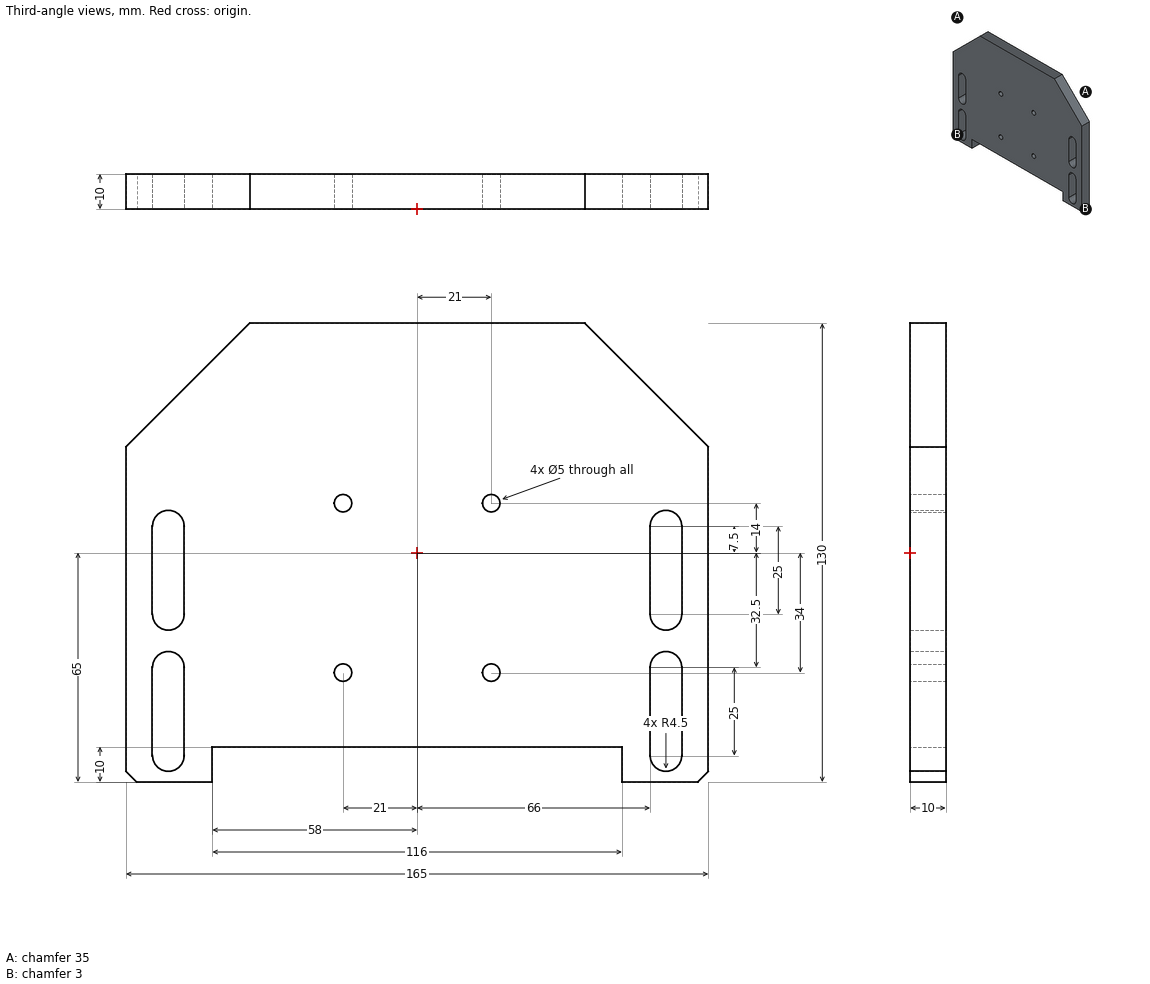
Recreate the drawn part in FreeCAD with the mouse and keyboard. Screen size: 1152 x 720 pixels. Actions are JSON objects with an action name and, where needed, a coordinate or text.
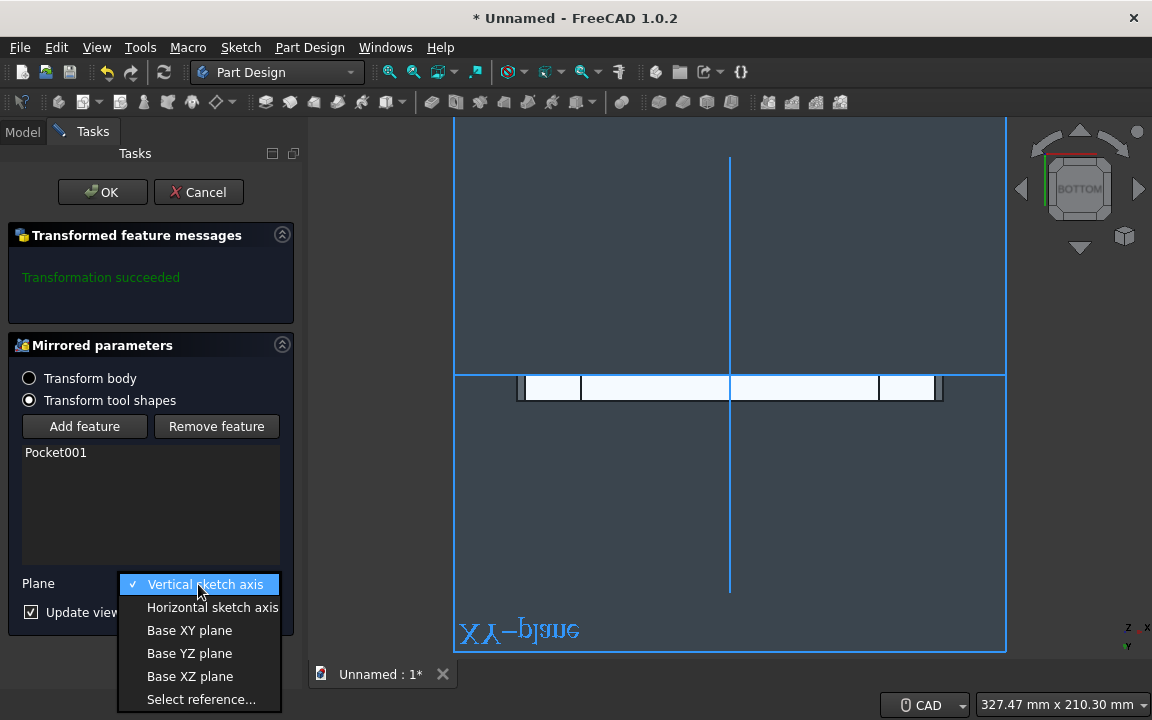
{"action": "left_click", "coordinate": [198, 654]}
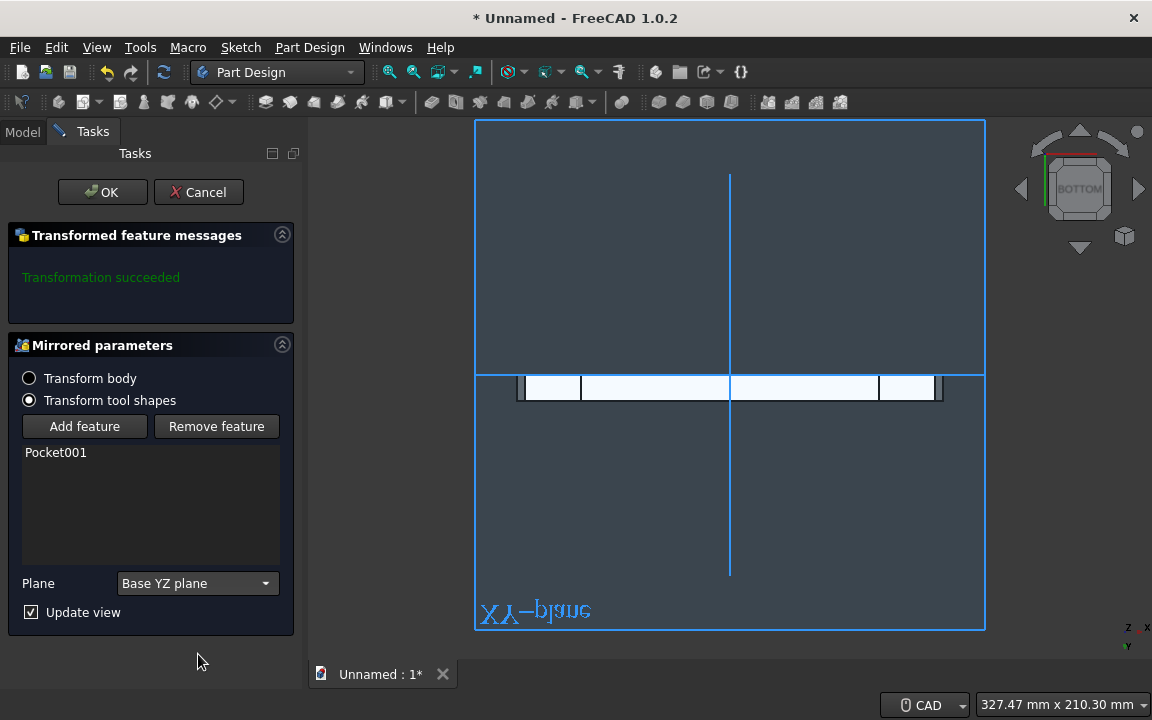
{"action": "left_click", "coordinate": [103, 192]}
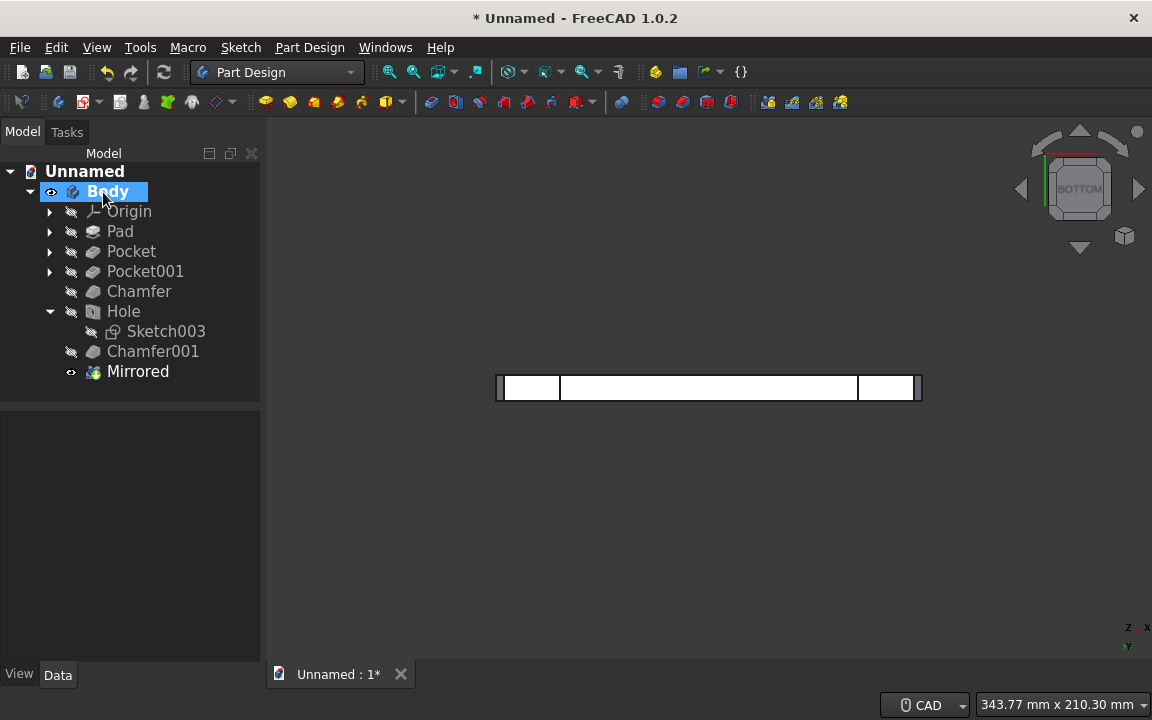
{"action": "key", "text": "0"}